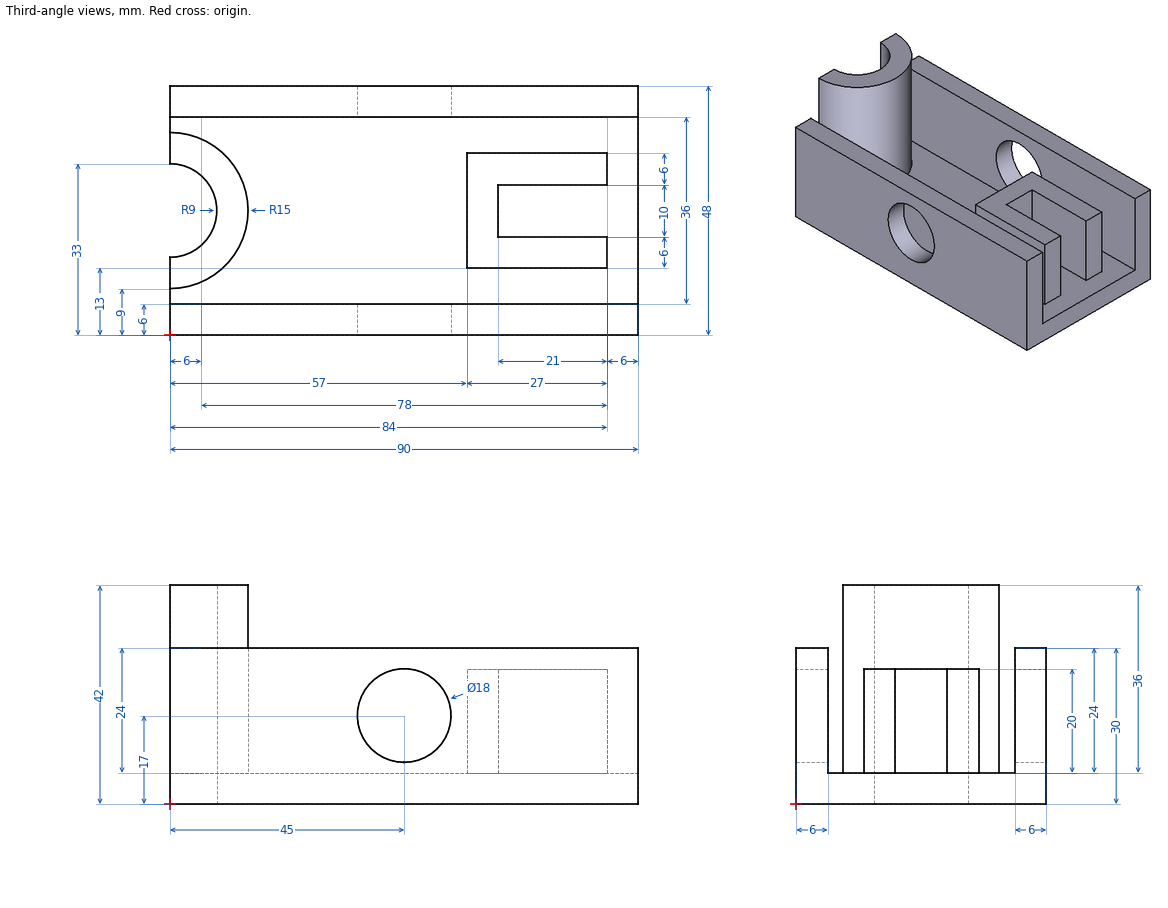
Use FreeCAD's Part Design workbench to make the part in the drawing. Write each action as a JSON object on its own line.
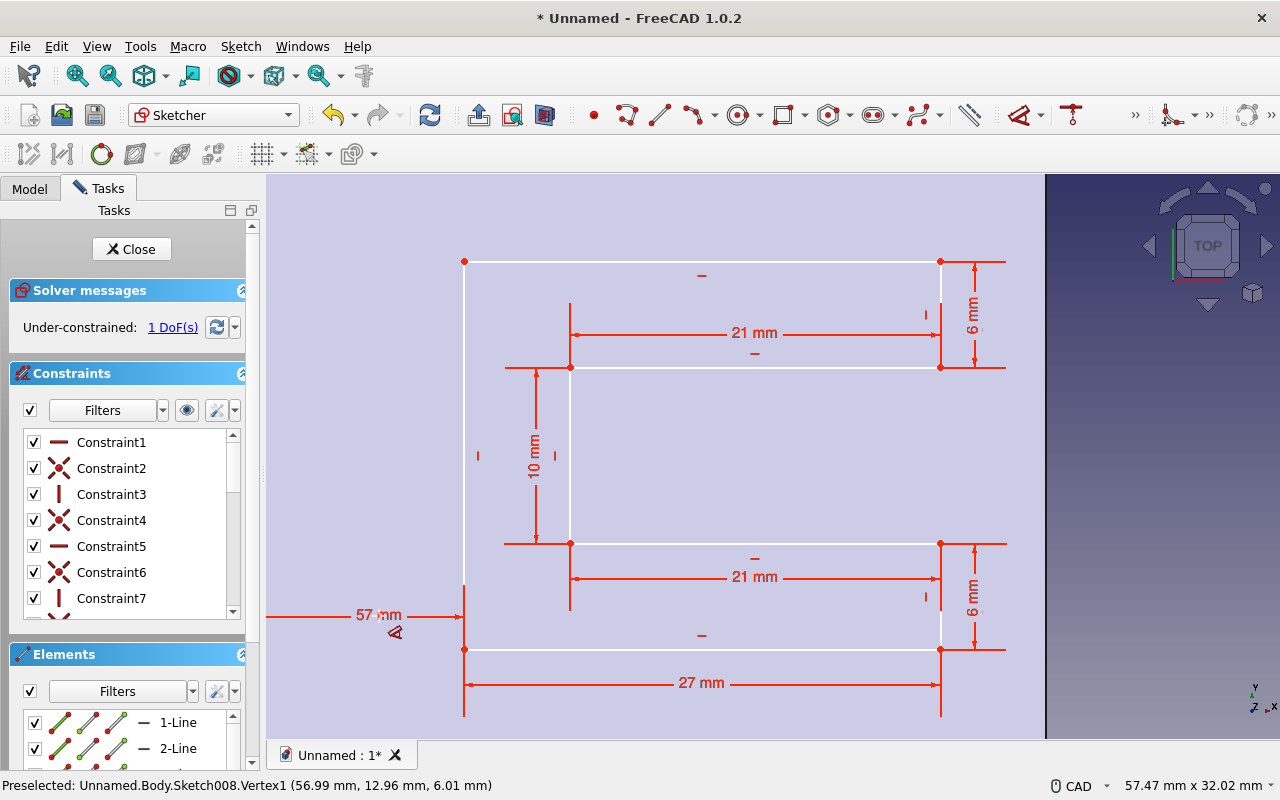
{"action": "left_click", "coordinate": [464, 650]}
{"action": "left_click", "coordinate": [498, 680]}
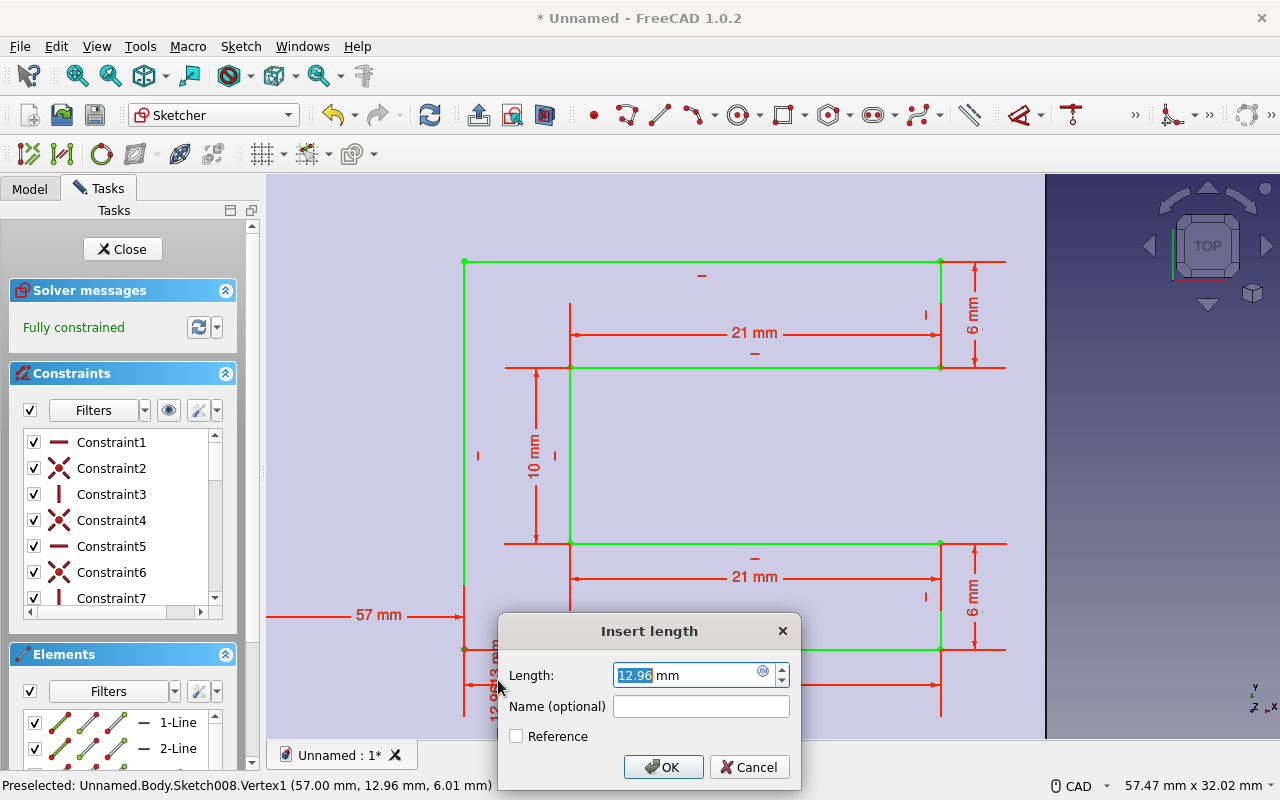
{"action": "type", "text": "13"}
{"action": "key", "text": "Return"}
{"action": "key", "text": "Escape"}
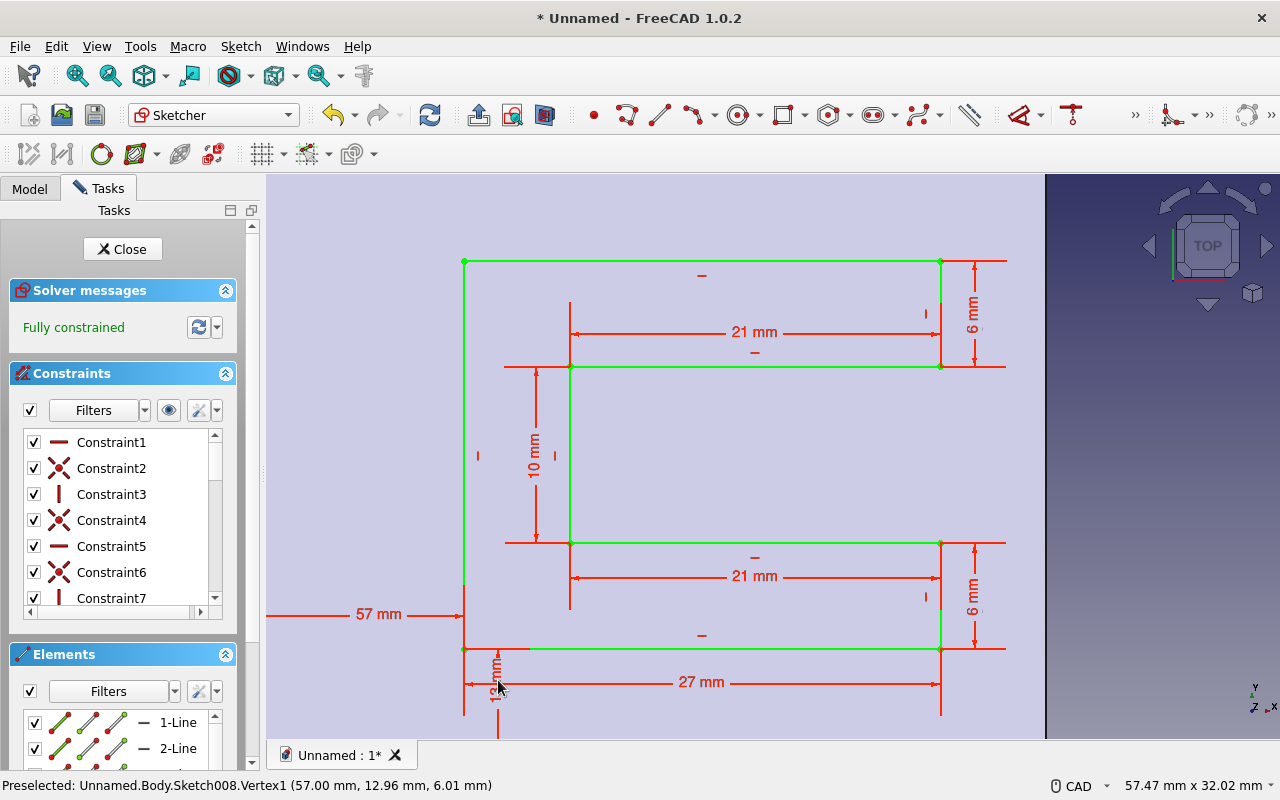
{"action": "left_click", "coordinate": [123, 249]}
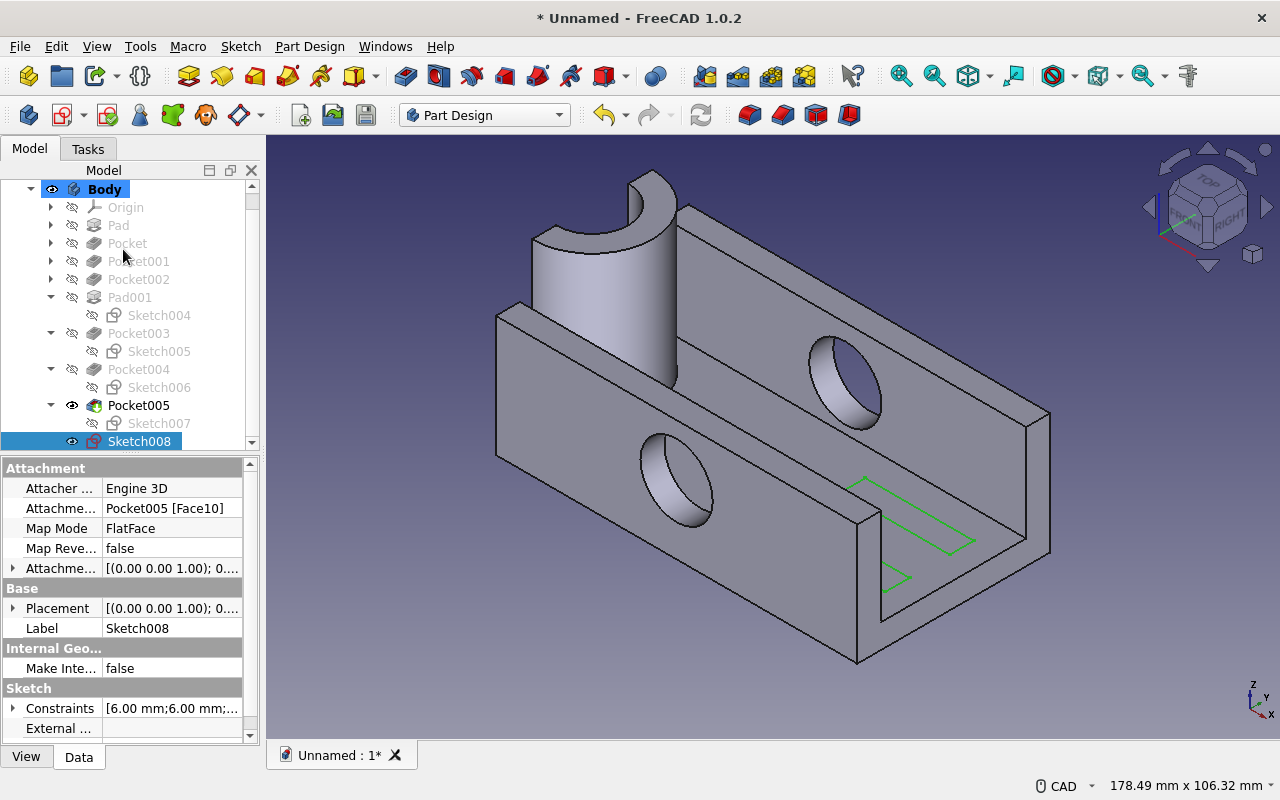
{"action": "left_click", "coordinate": [189, 76]}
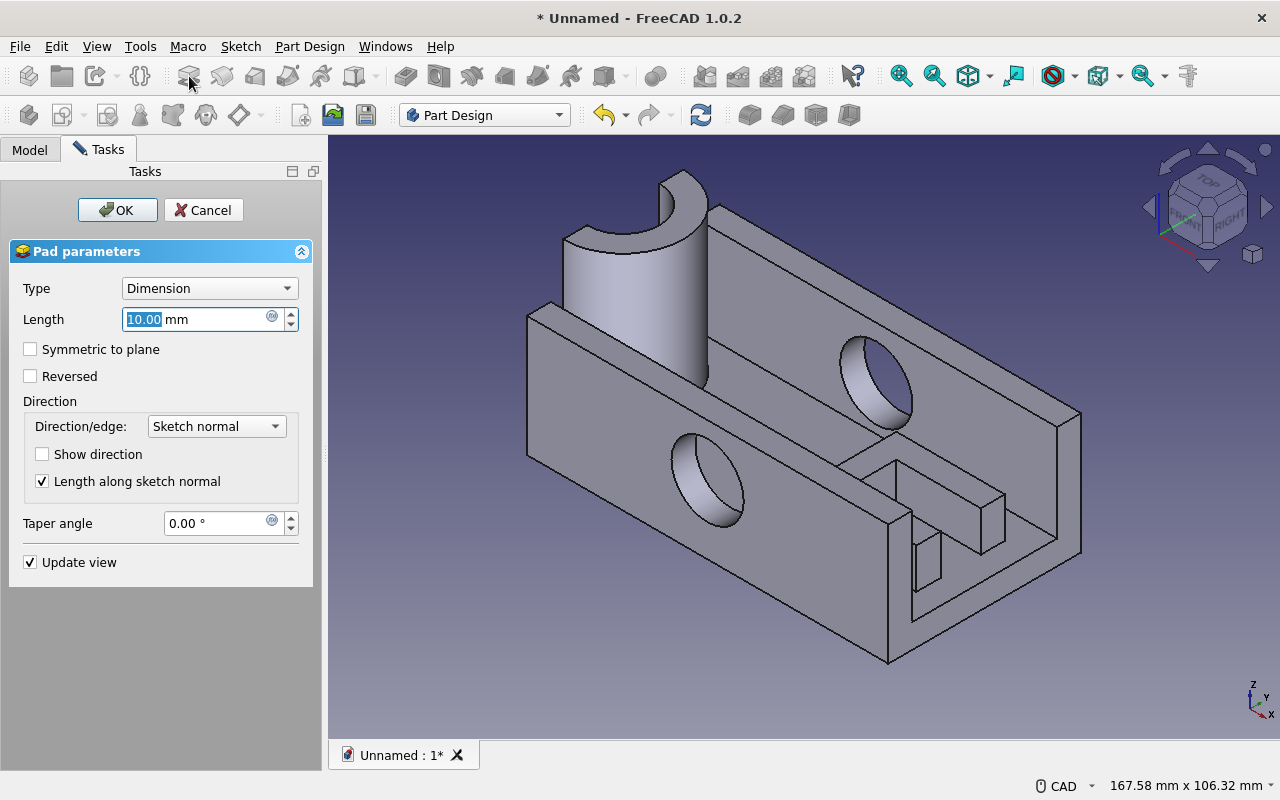
{"action": "type", "text": "20"}
{"action": "key", "text": "Tab"}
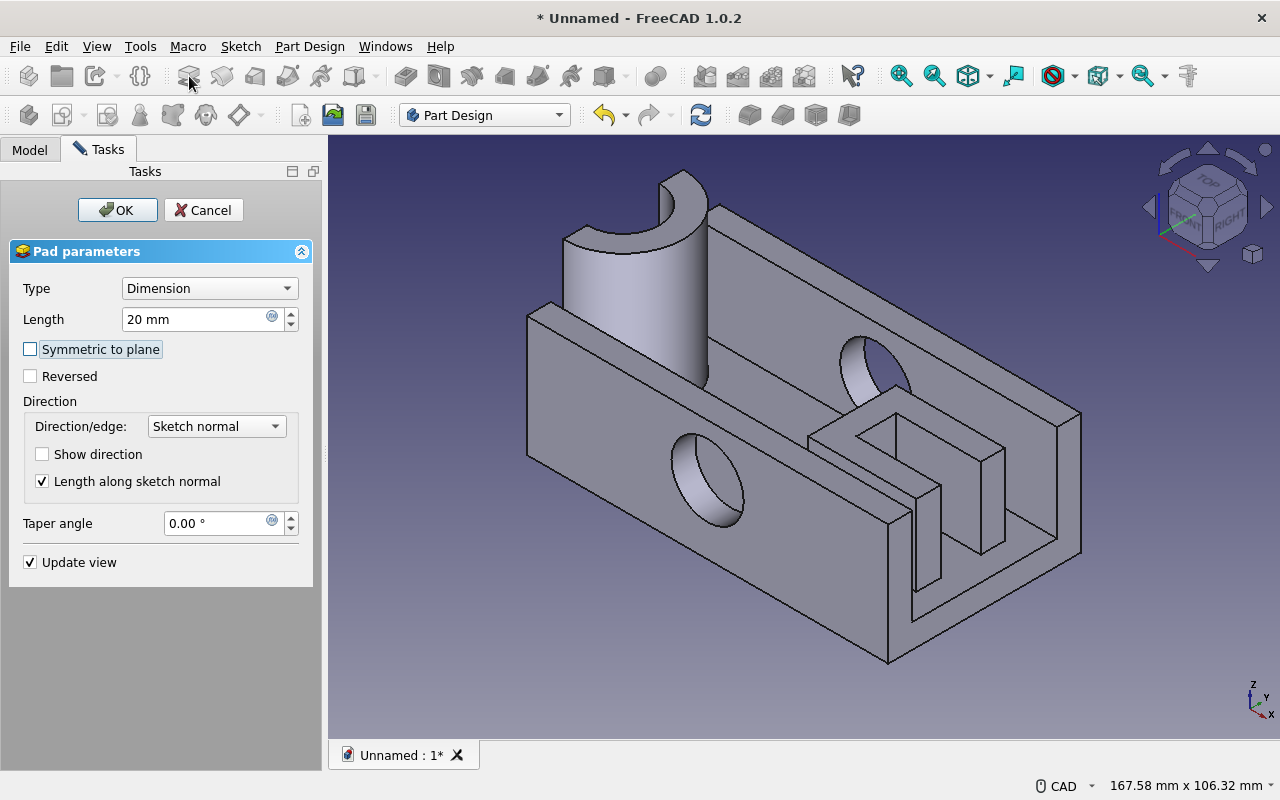
{"action": "left_click", "coordinate": [118, 210]}